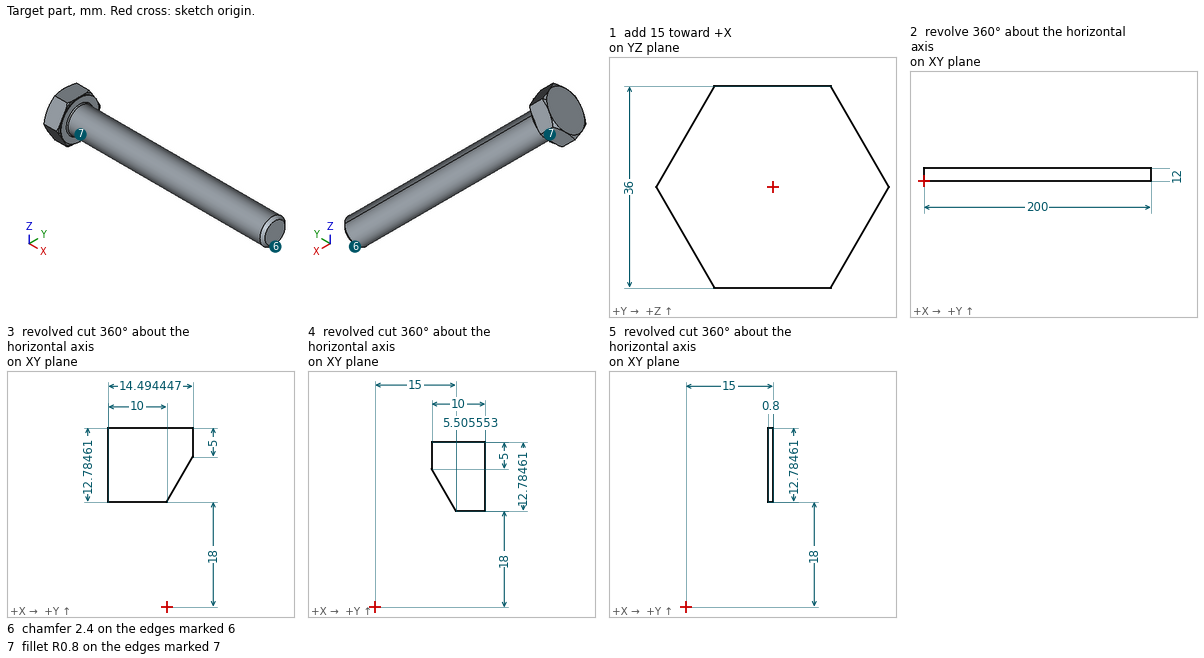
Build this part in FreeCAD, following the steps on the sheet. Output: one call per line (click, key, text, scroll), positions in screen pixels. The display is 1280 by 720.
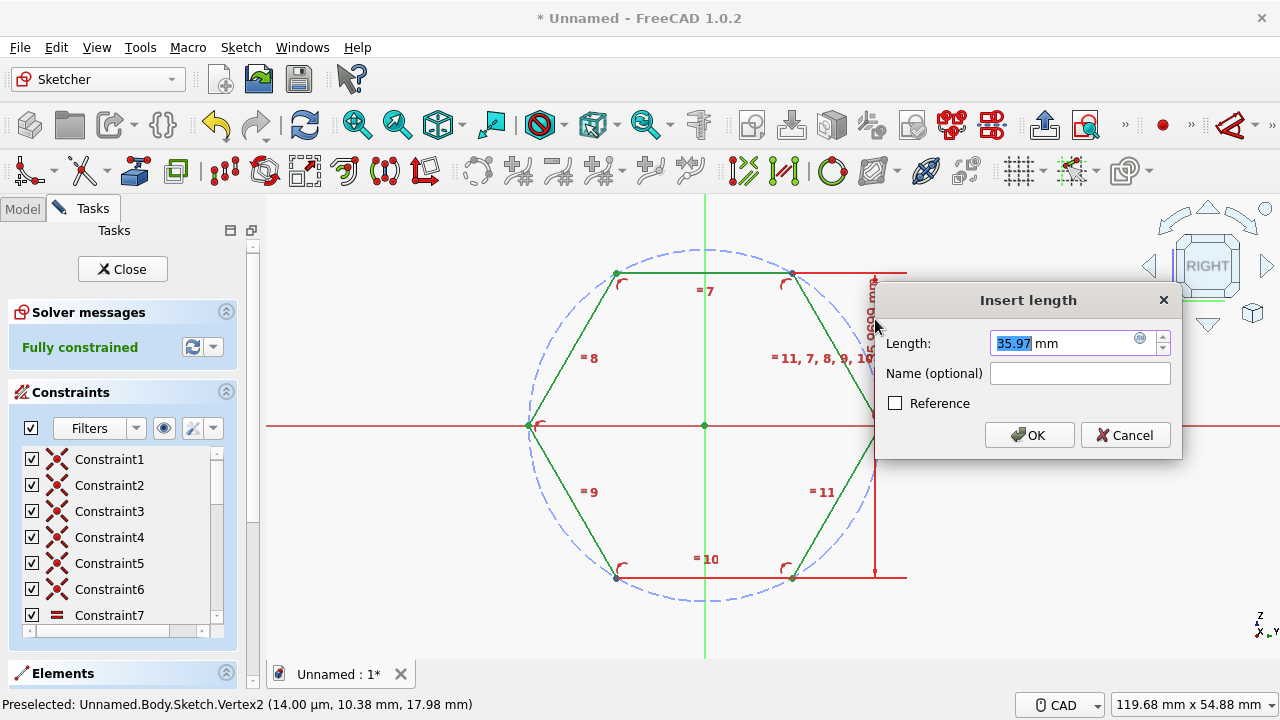
text(36)
key(Return)
key(Escape)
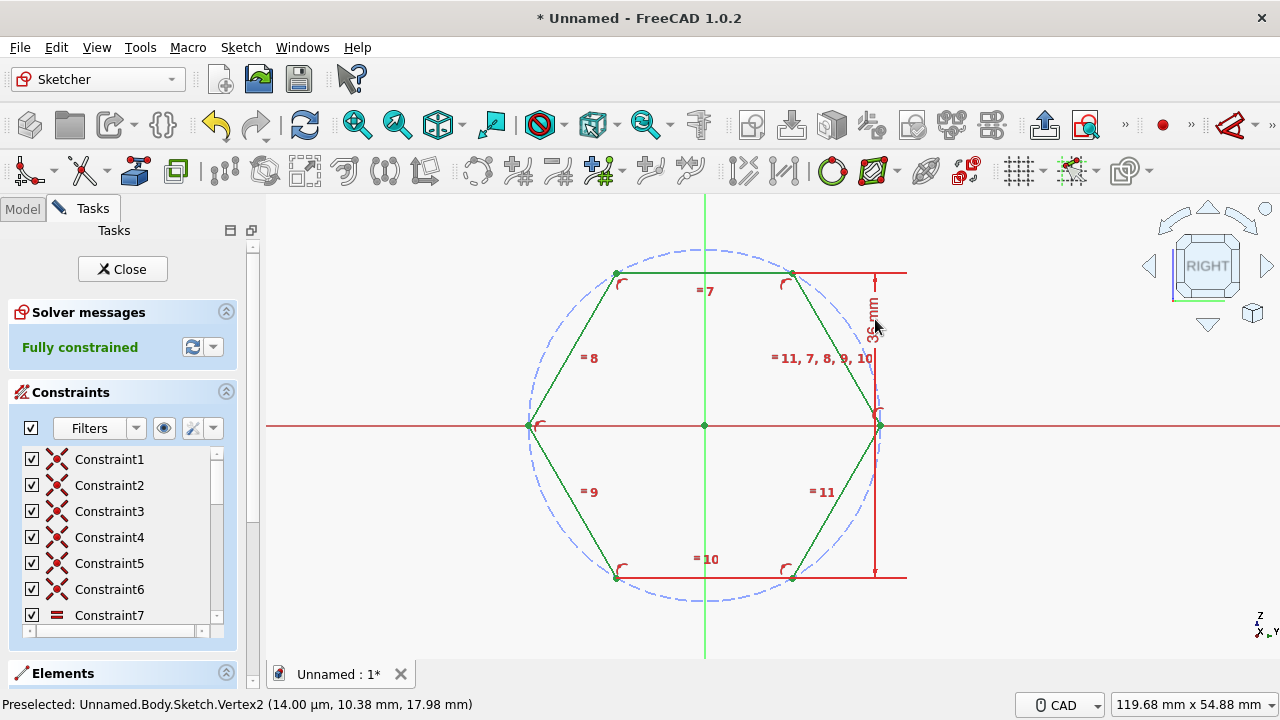
click(123, 269)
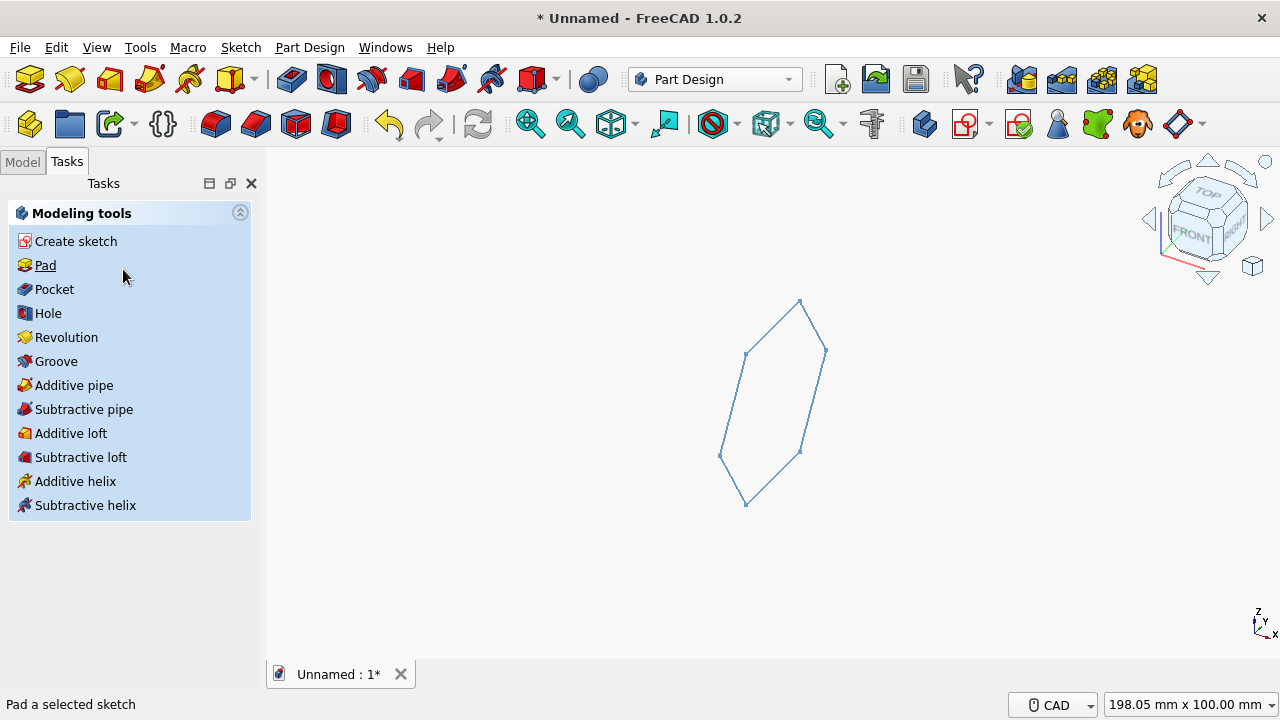
click(30, 80)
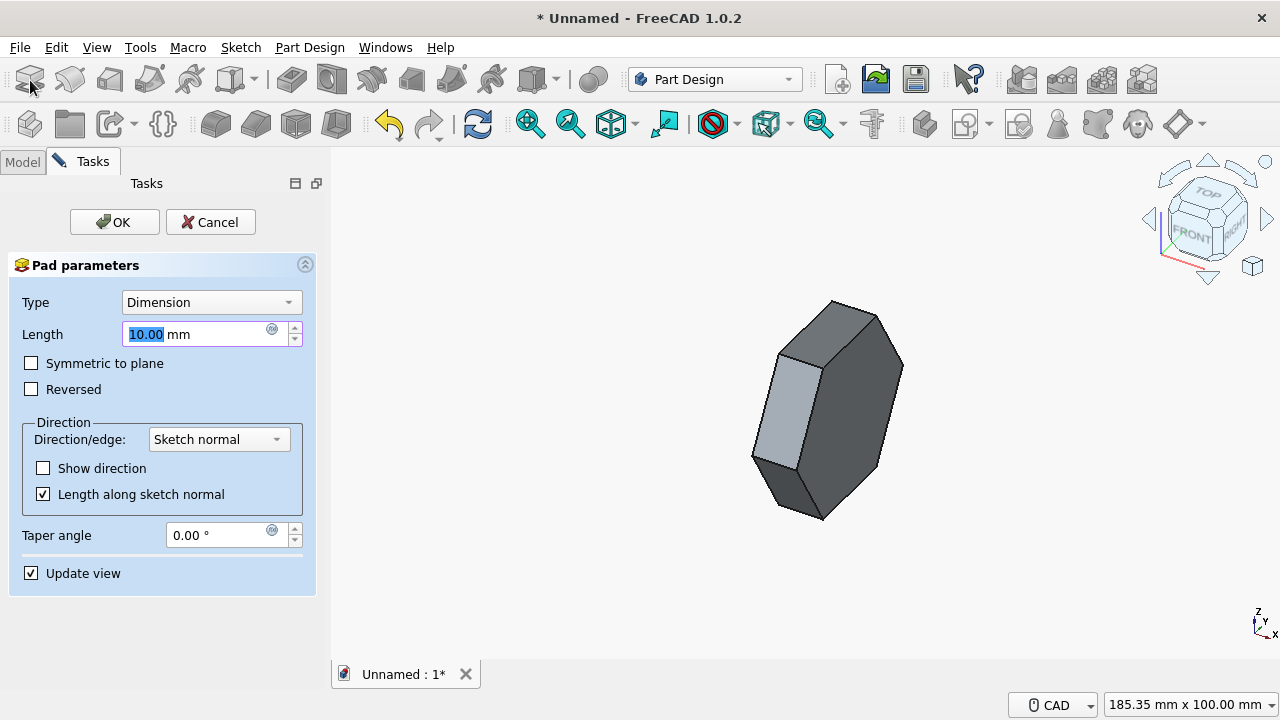
text(15)
key(Tab)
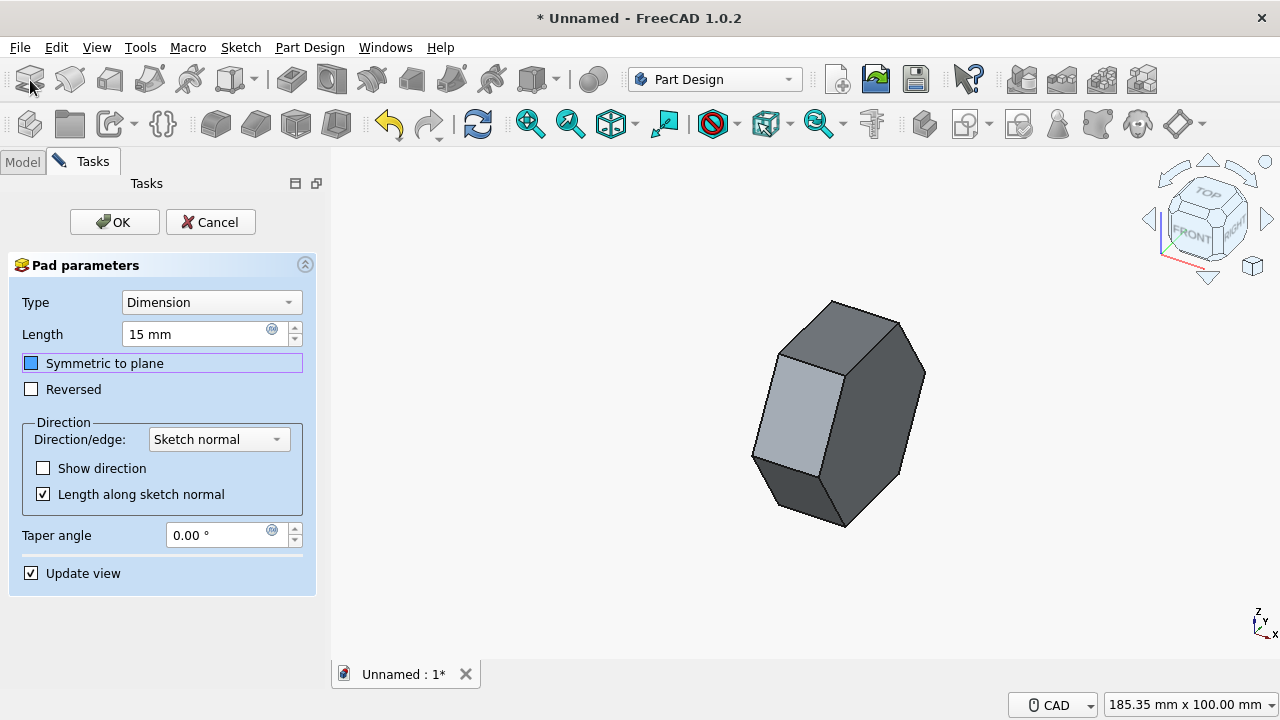
click(115, 222)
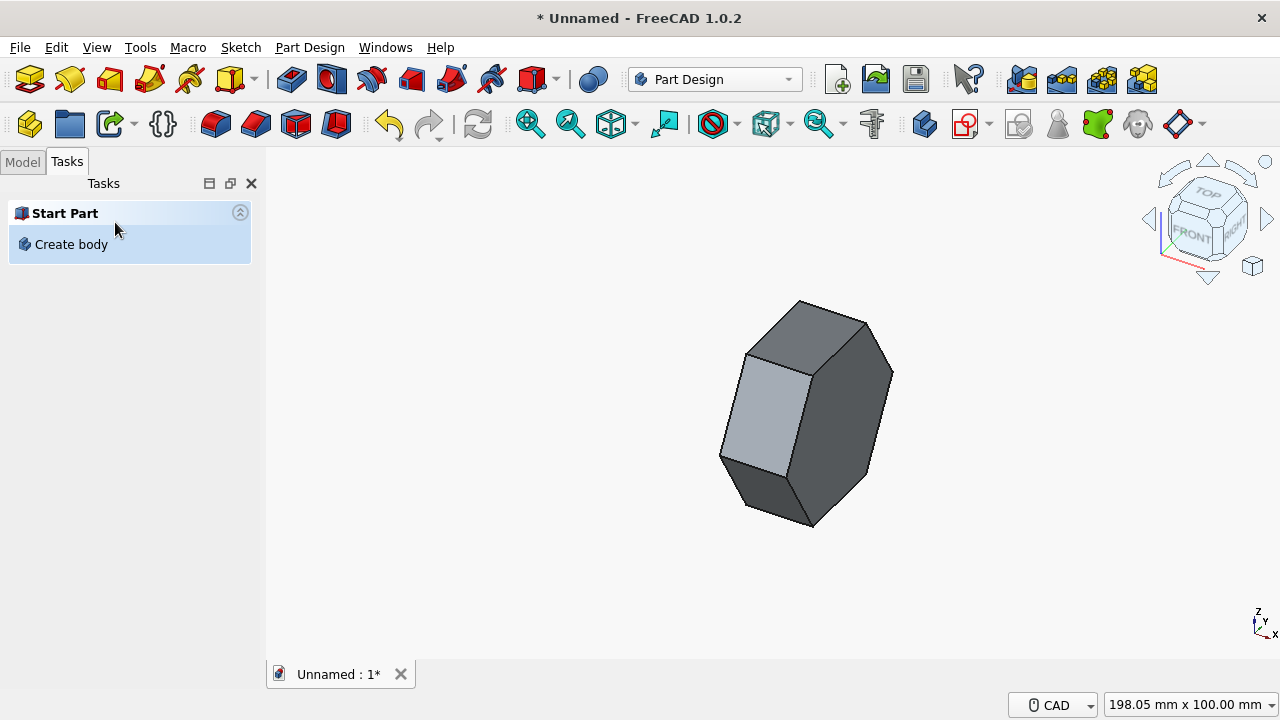
click(966, 124)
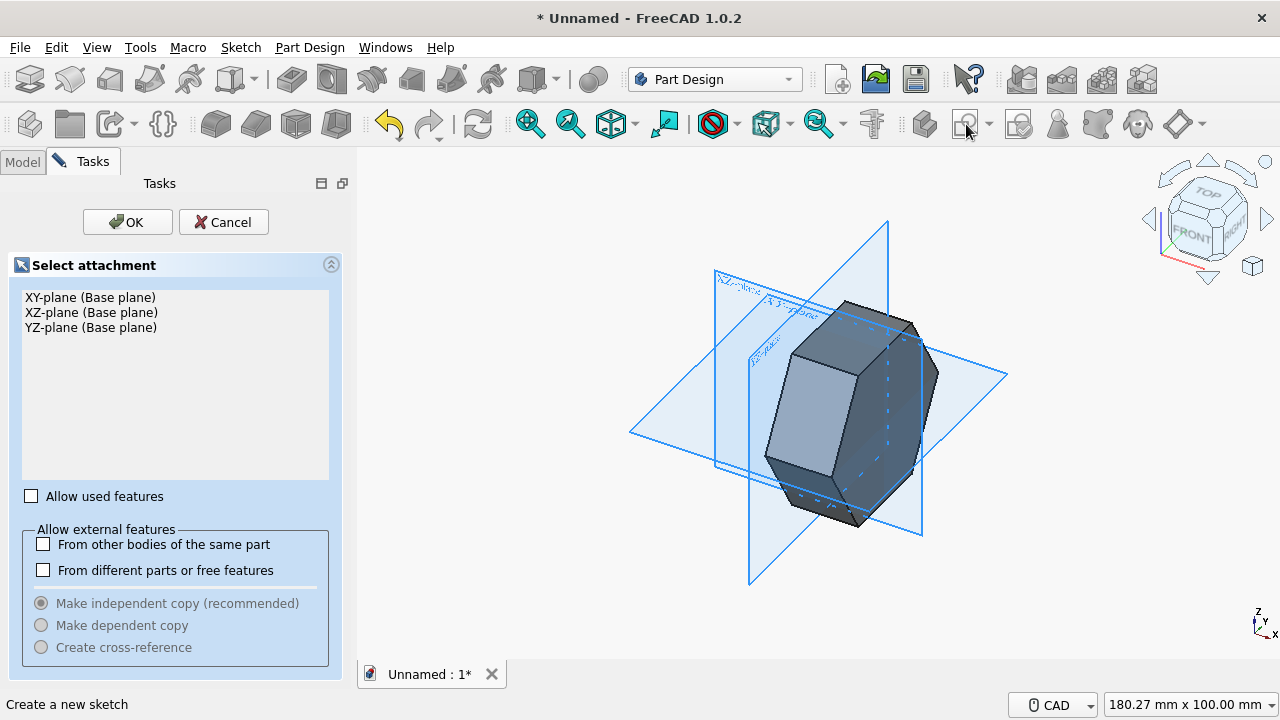
click(82, 298)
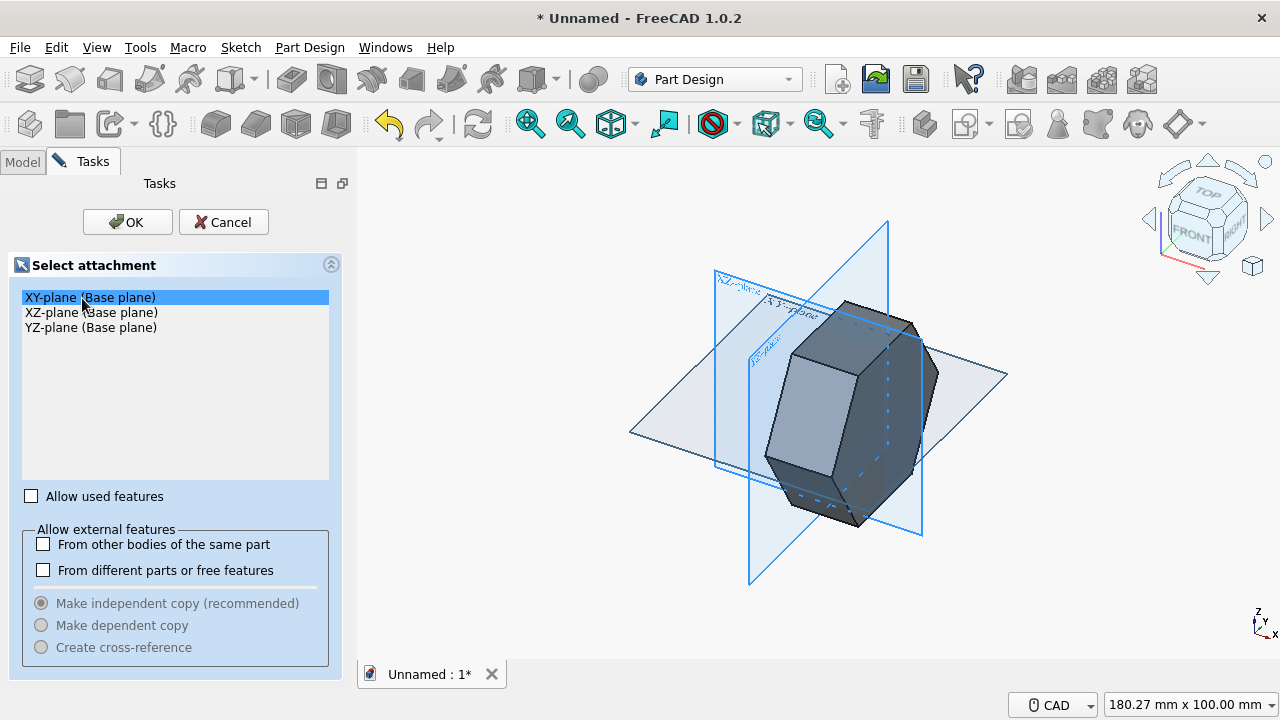
click(128, 222)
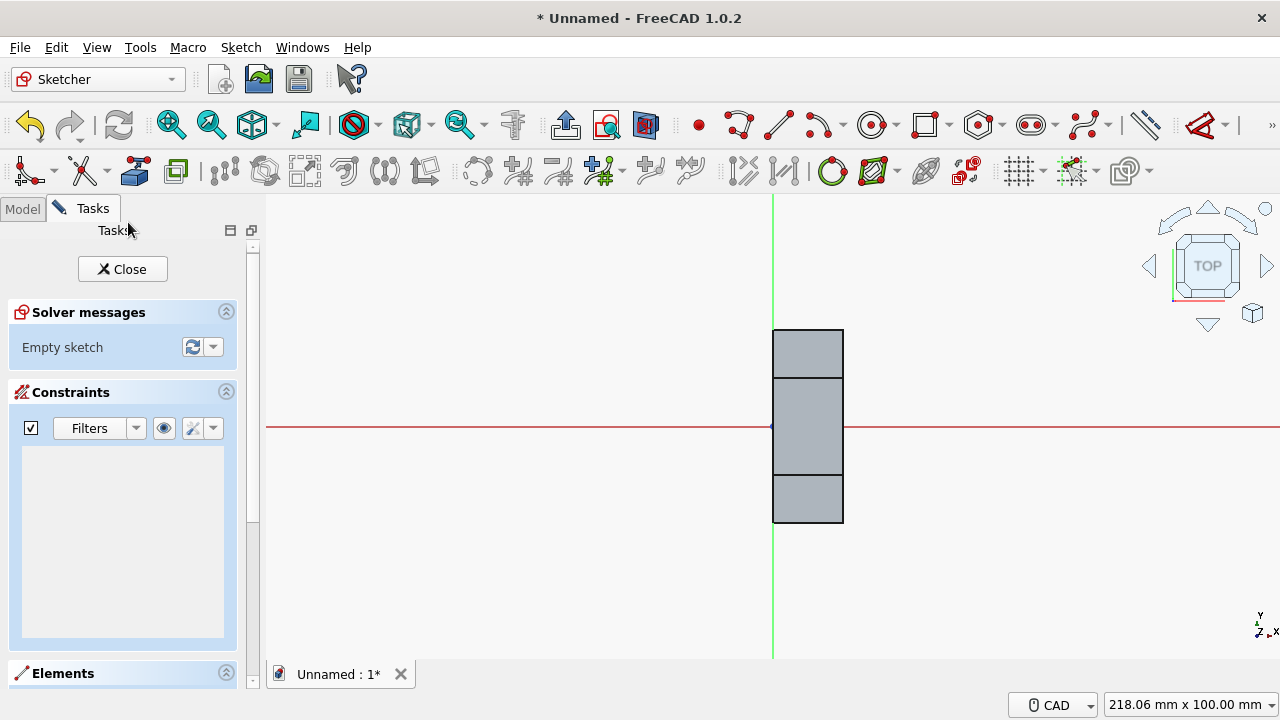
click(646, 126)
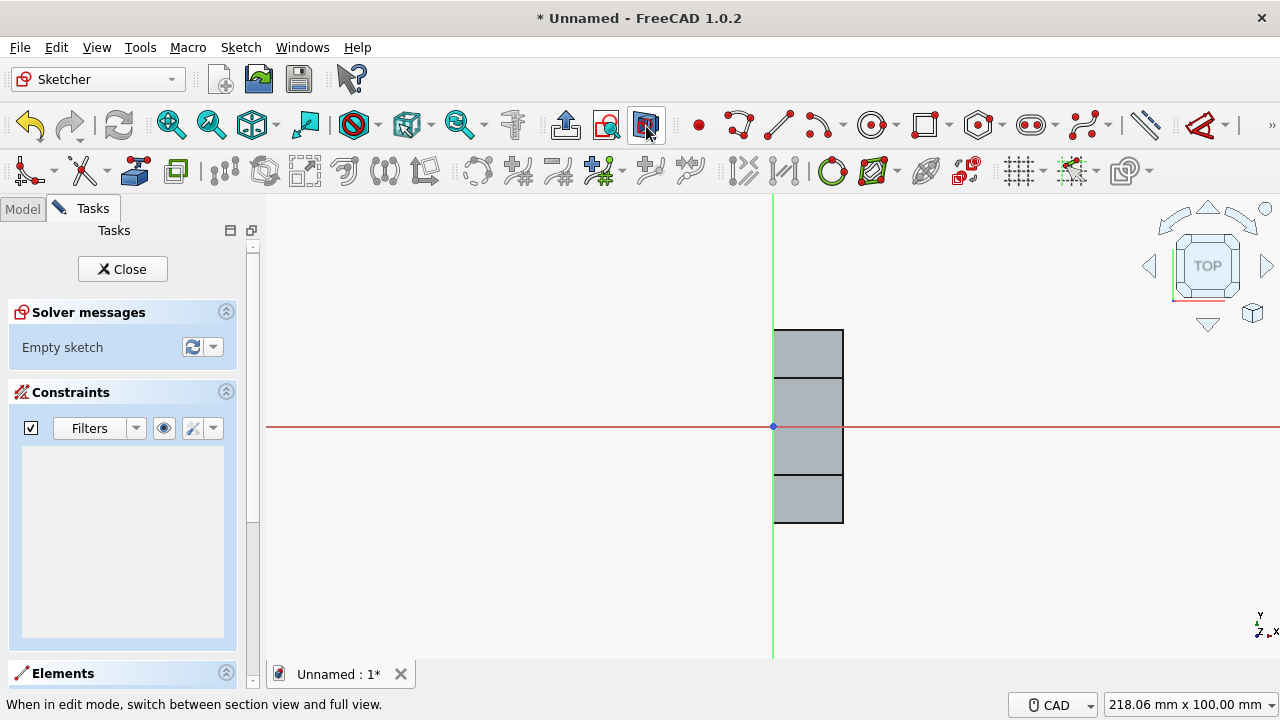
scroll(294, 460, down, 3)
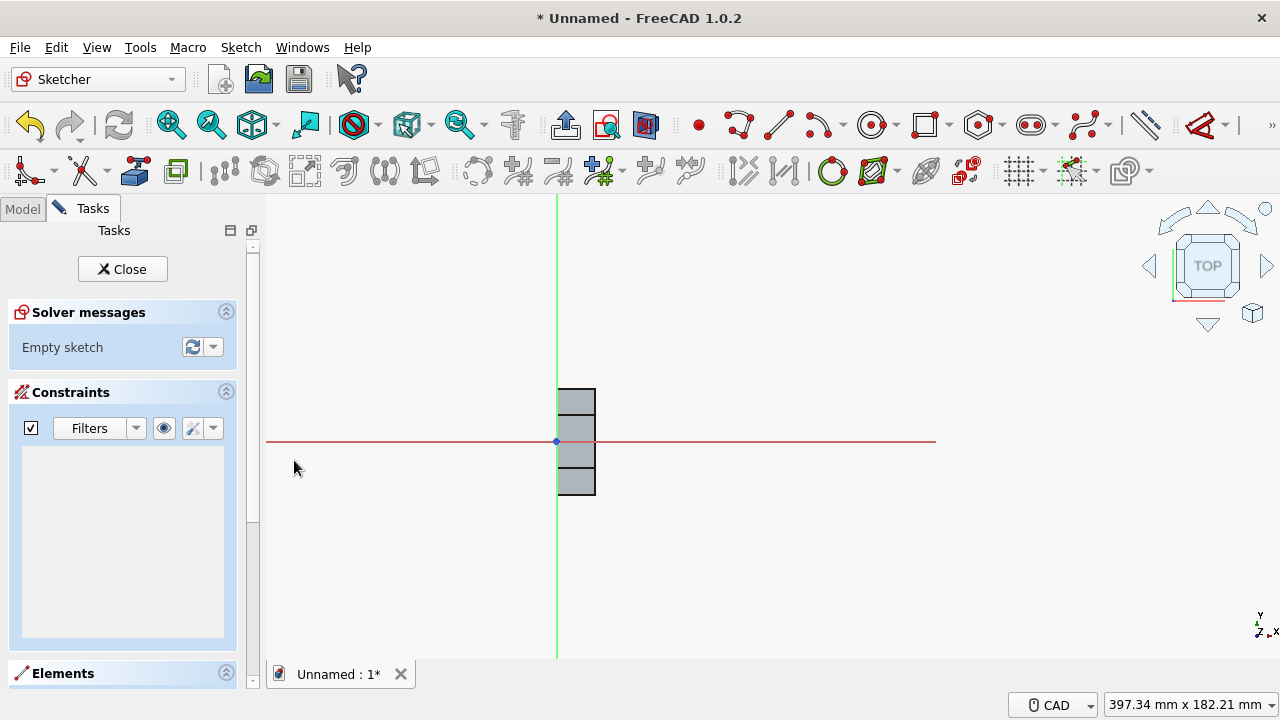
key(g)
key(r)